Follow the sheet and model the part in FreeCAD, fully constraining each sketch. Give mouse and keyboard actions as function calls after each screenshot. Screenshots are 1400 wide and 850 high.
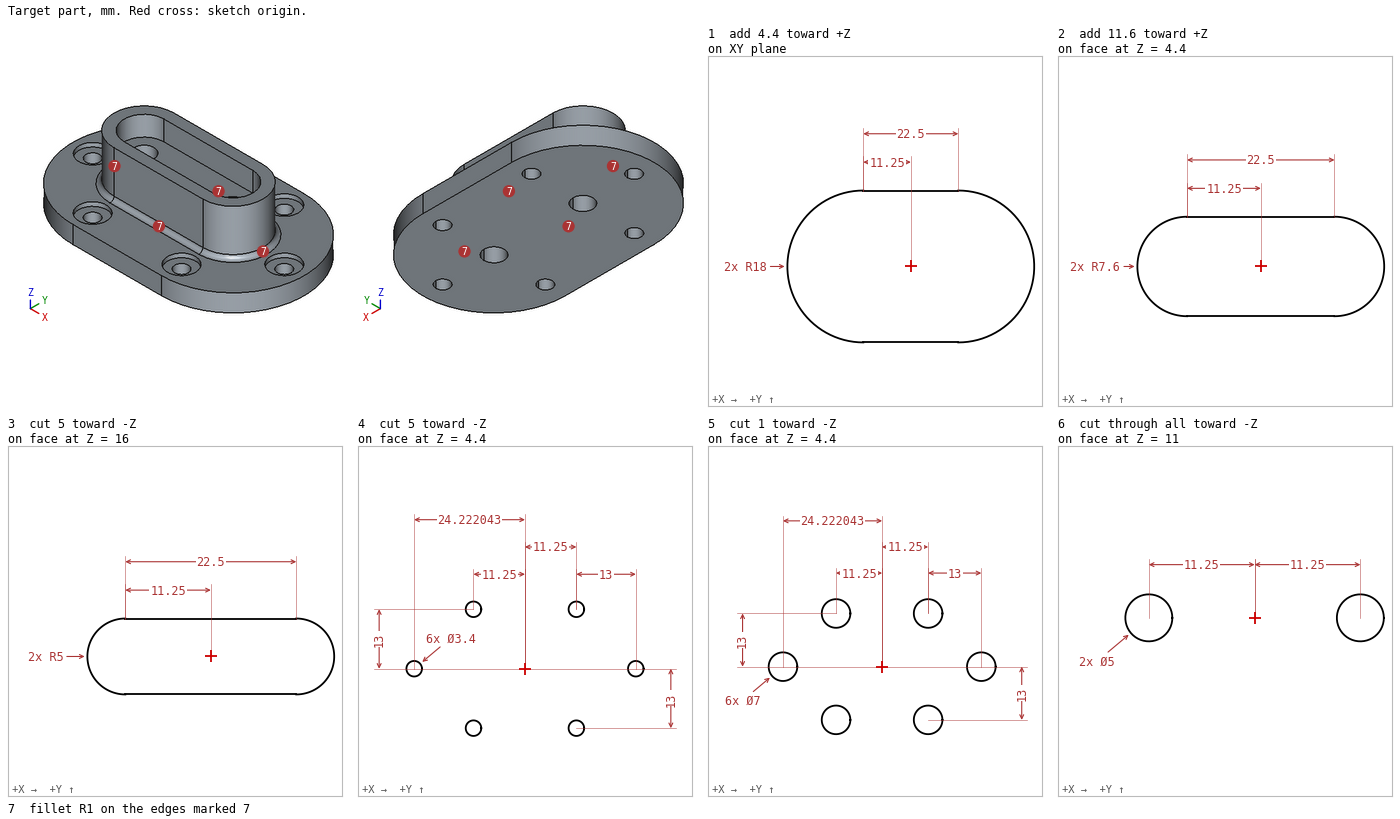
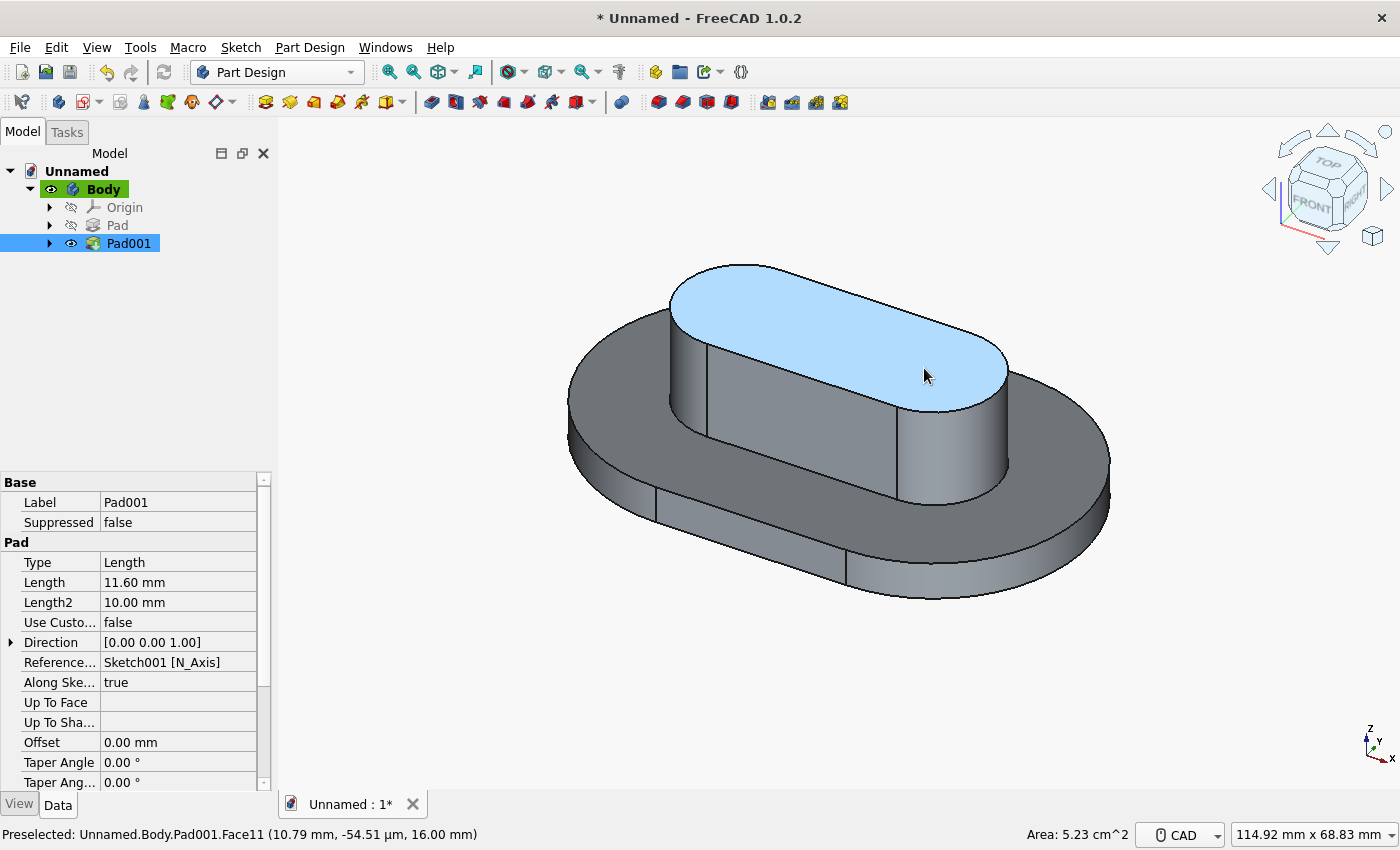
click(84, 102)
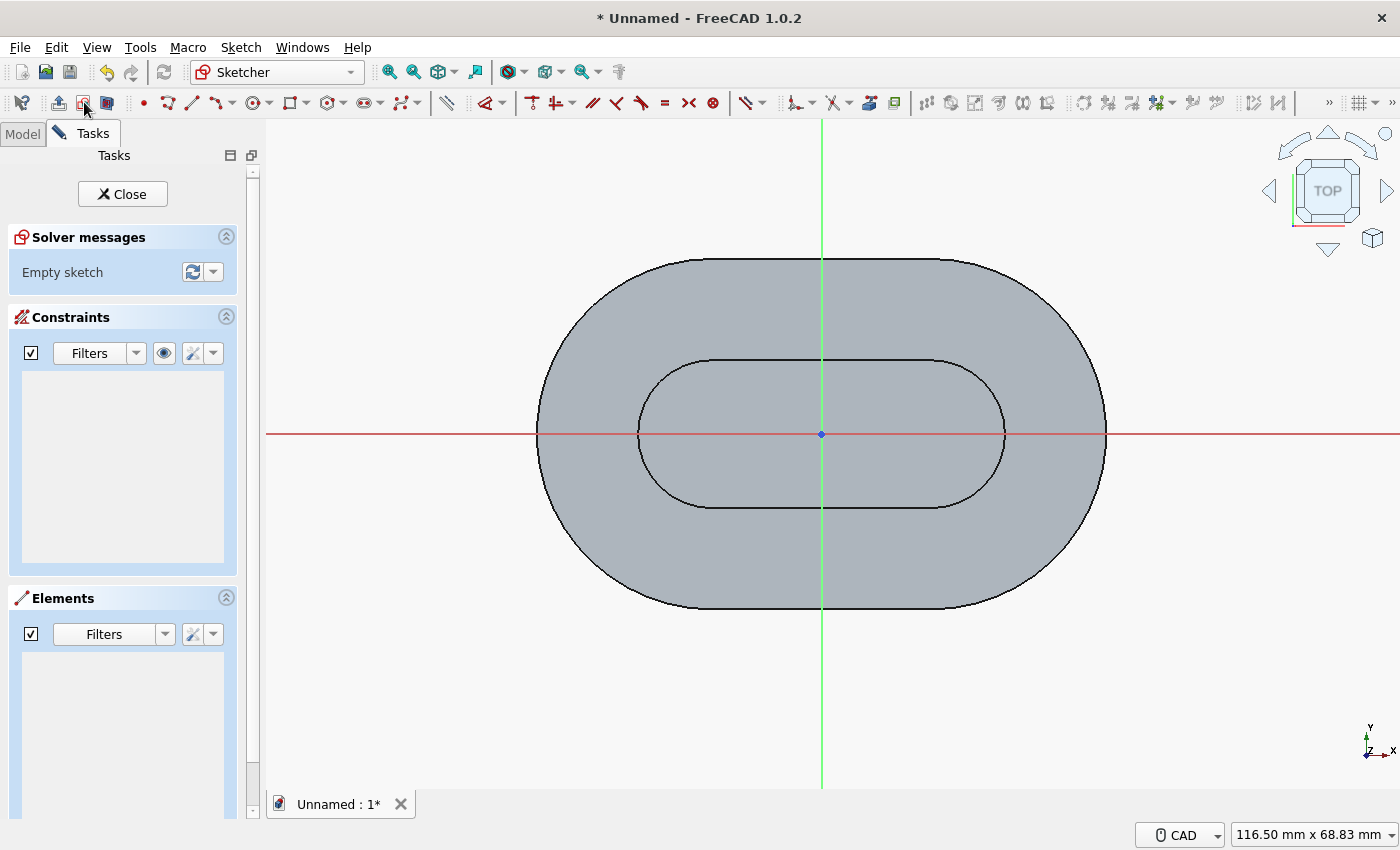
scroll(868, 418, up, 4)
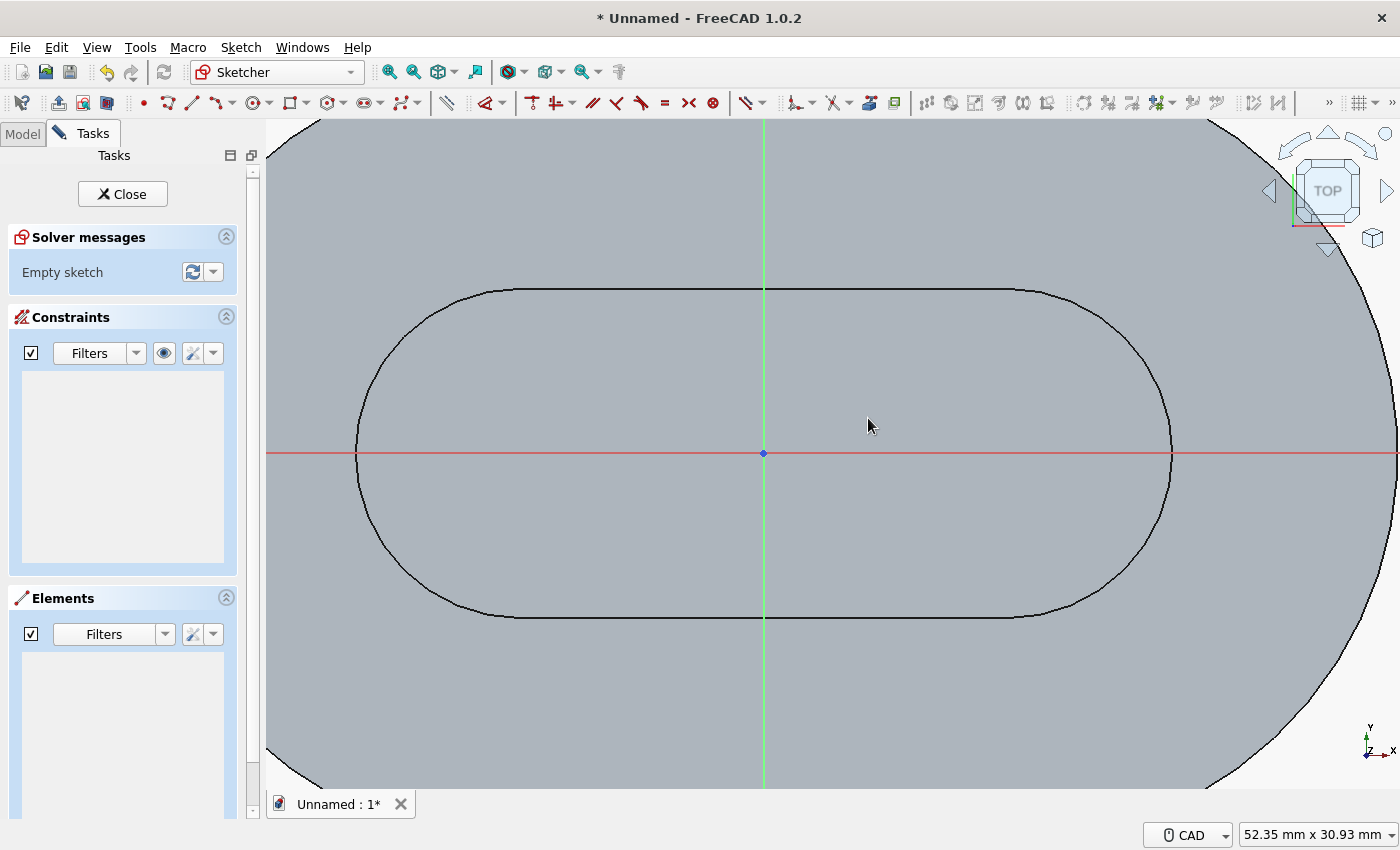
click(364, 104)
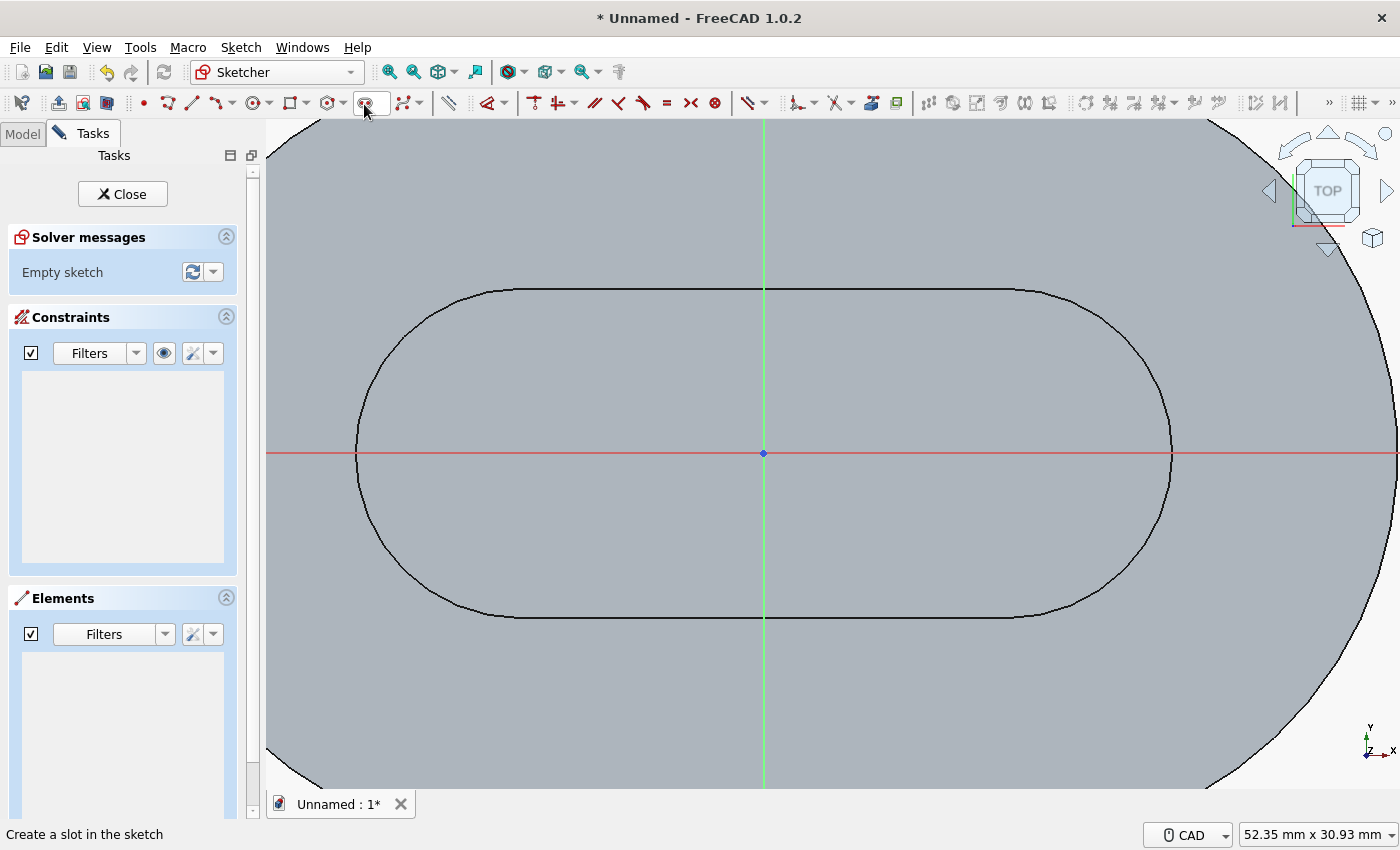
click(520, 453)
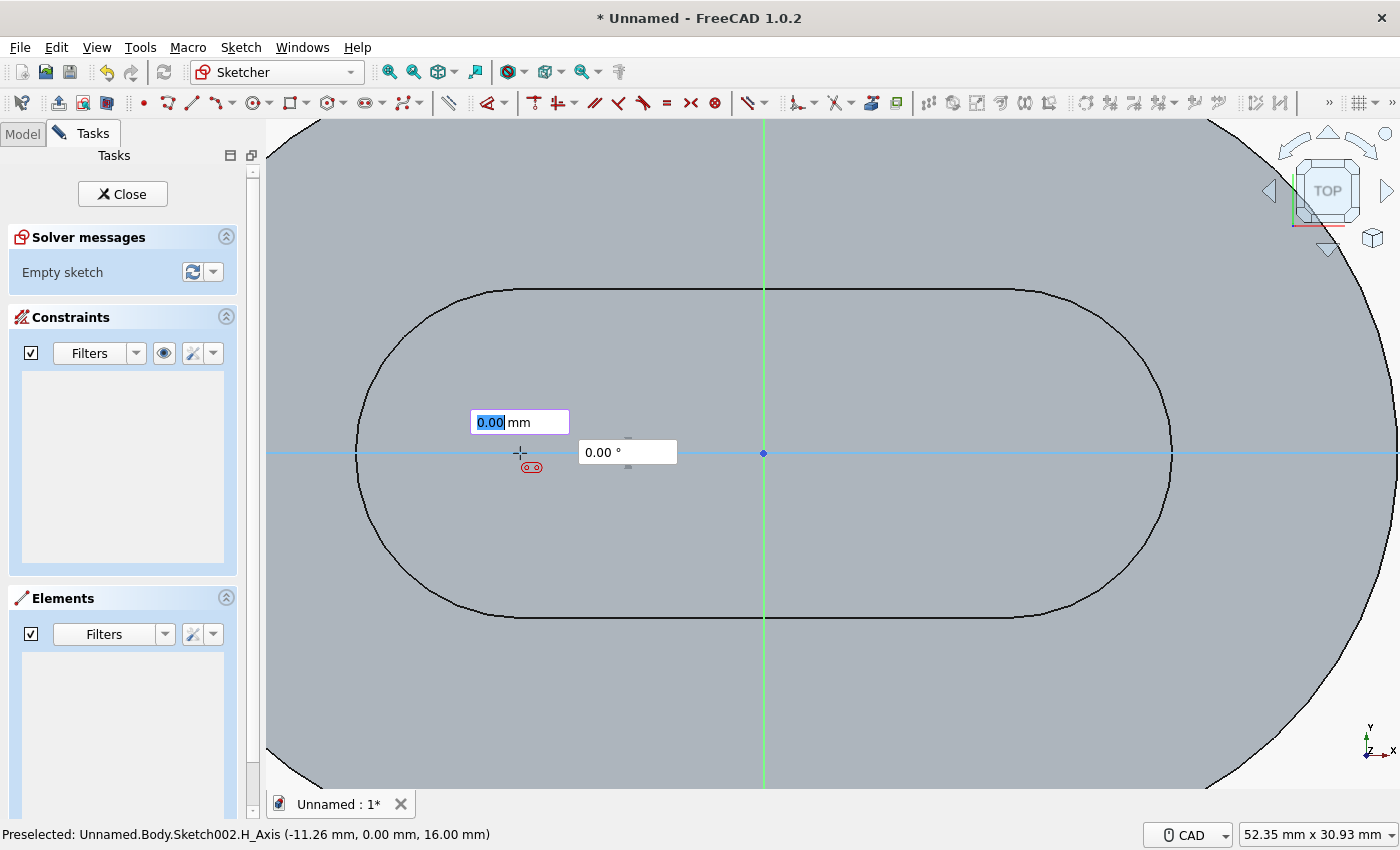
click(1008, 444)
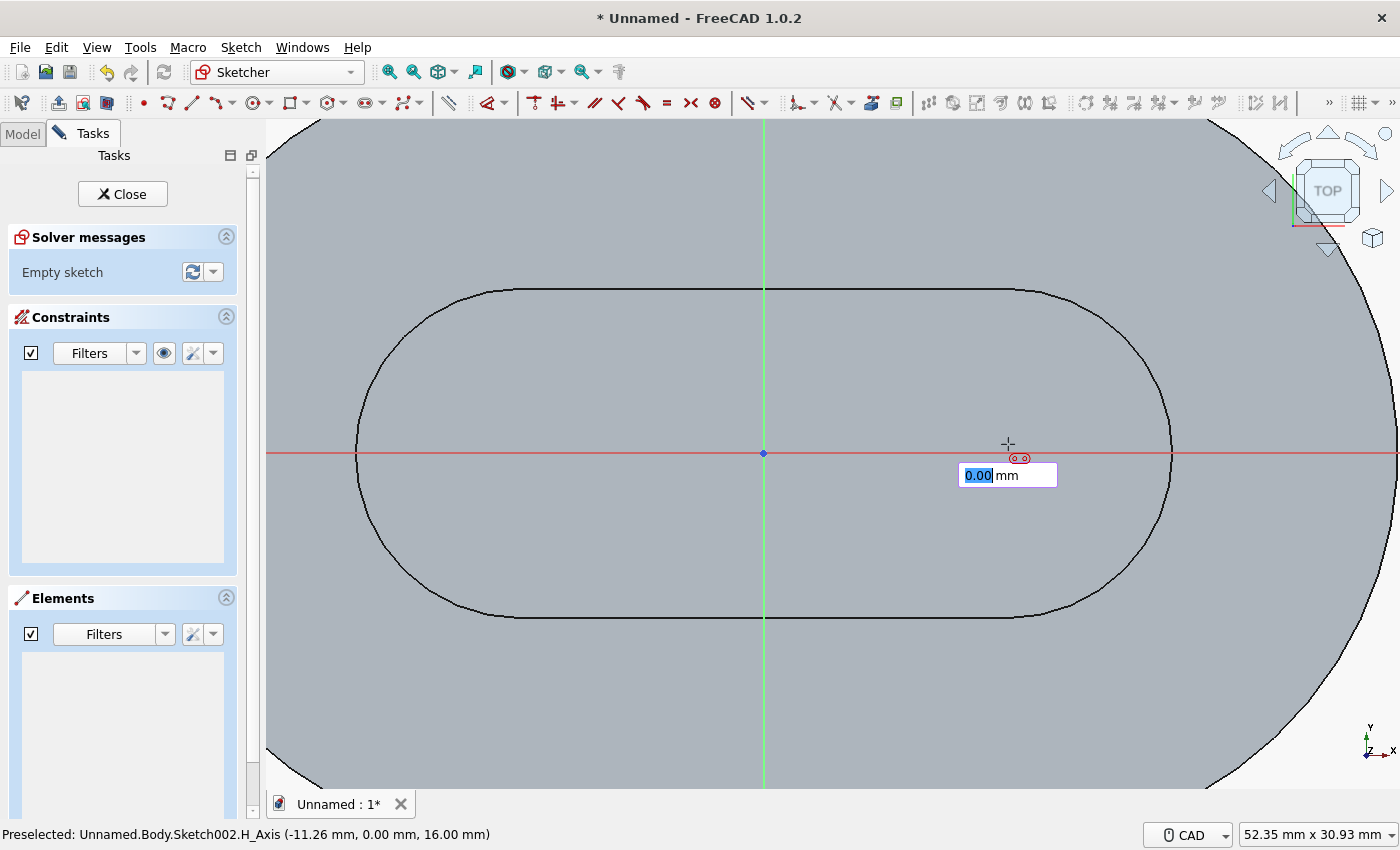
click(837, 345)
key(Escape)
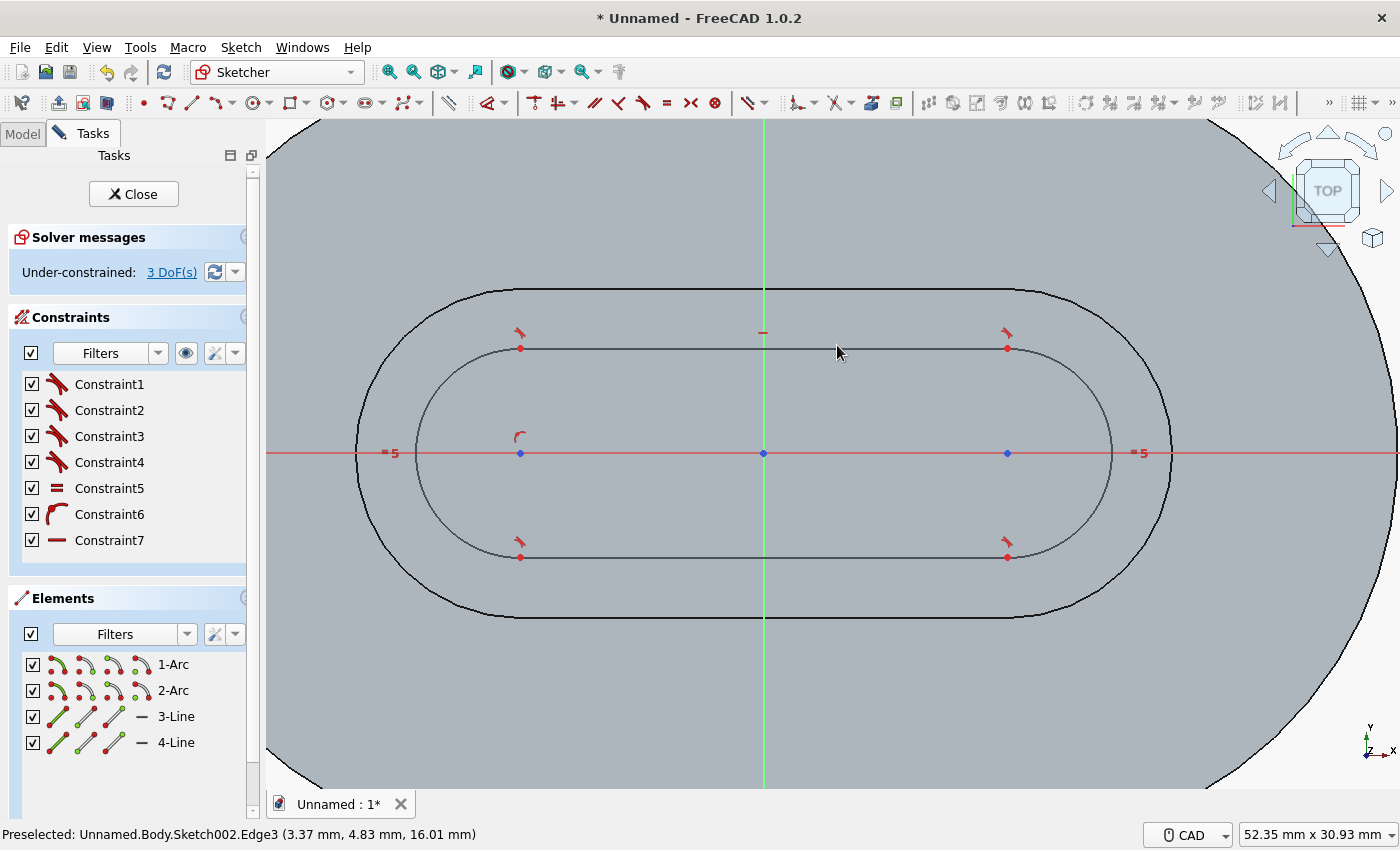
click(488, 104)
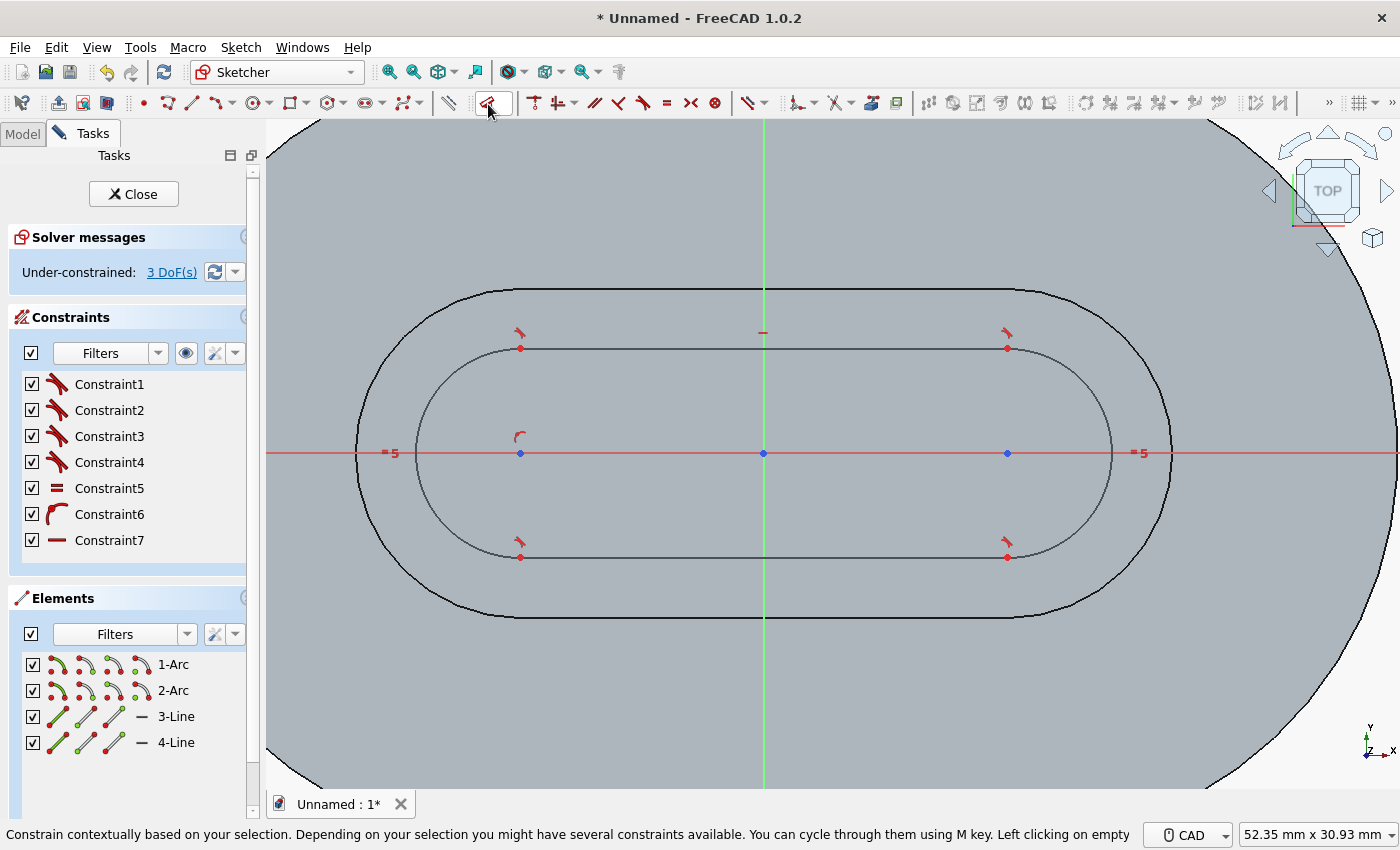
click(436, 392)
click(410, 373)